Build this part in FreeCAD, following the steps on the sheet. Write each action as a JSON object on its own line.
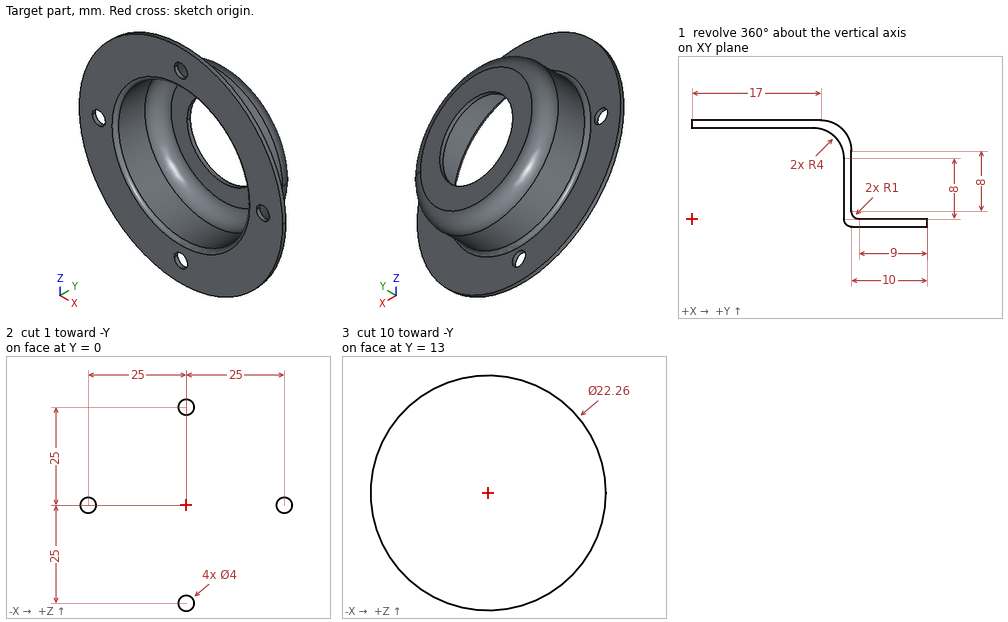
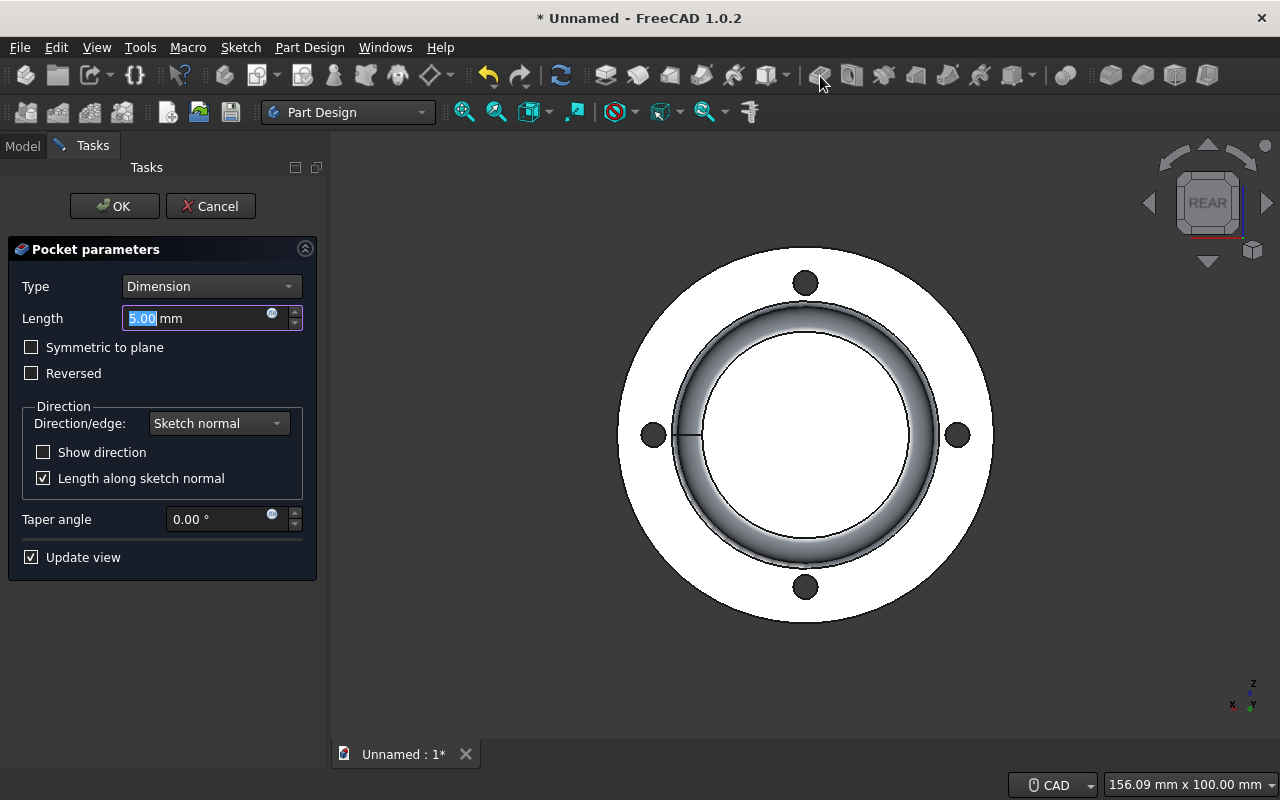
{"action": "type", "text": "1"}
{"action": "key", "text": "Tab"}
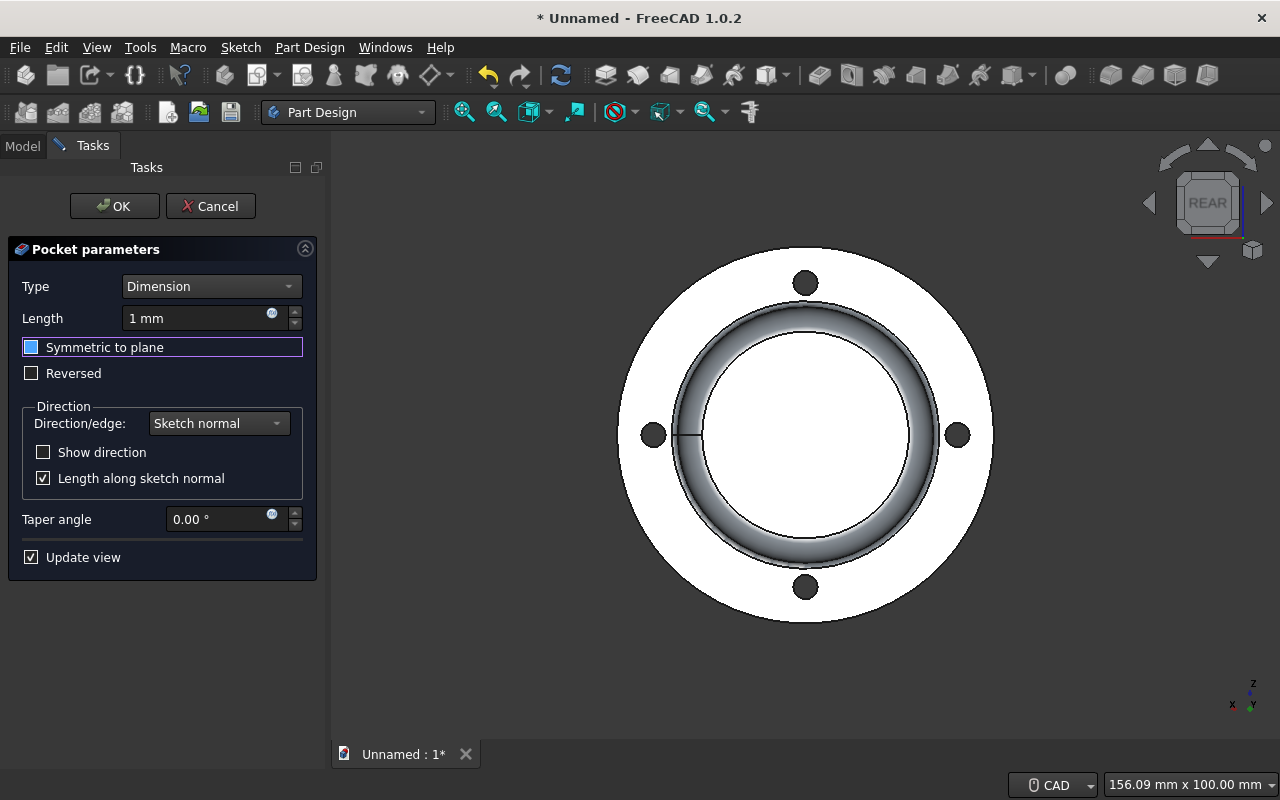
{"action": "left_click", "coordinate": [115, 206]}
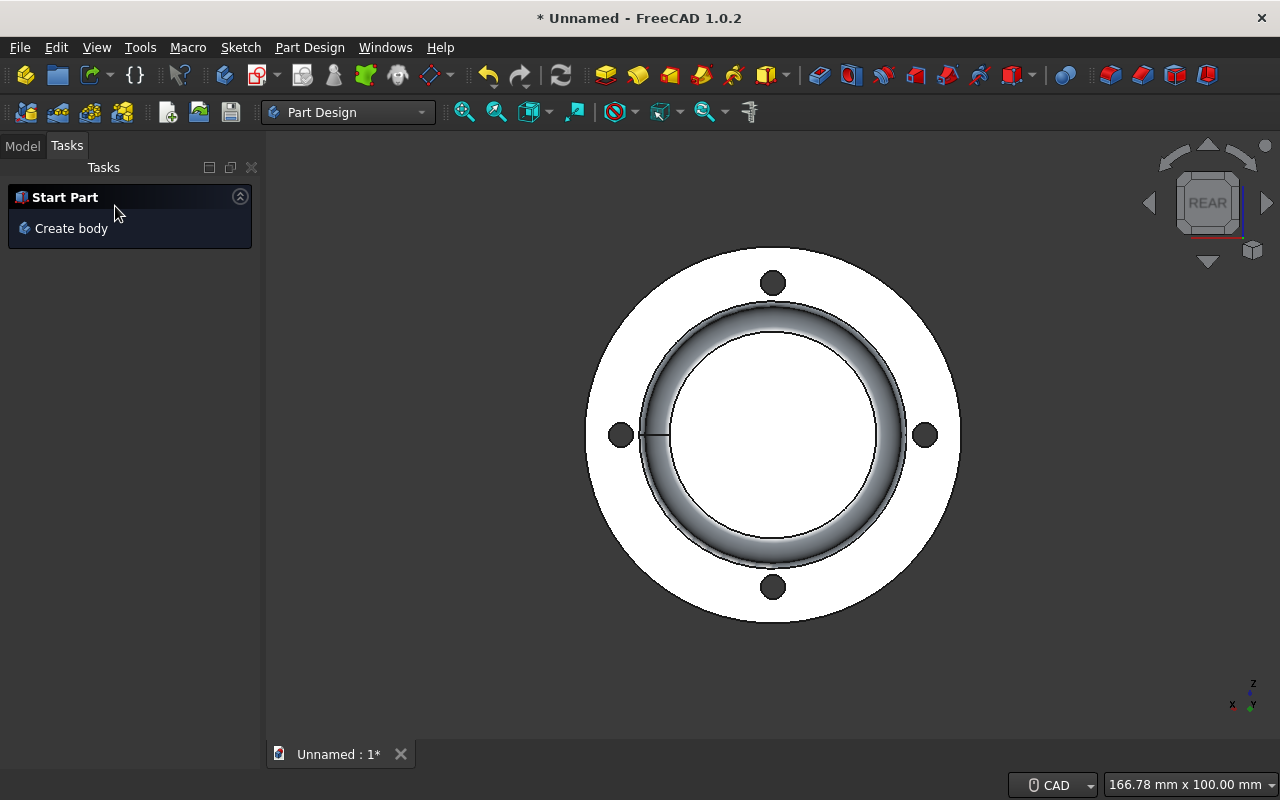
{"action": "left_click", "coordinate": [773, 434]}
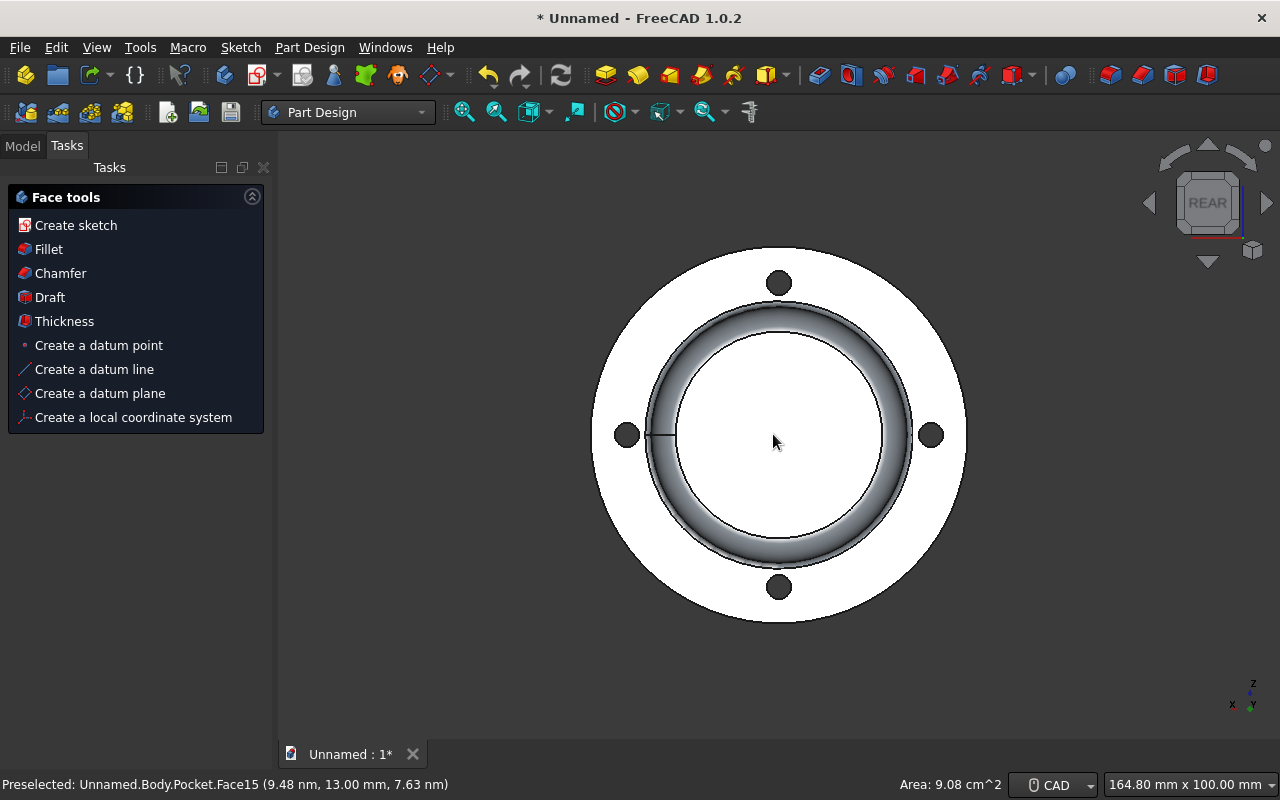
{"action": "left_click", "coordinate": [258, 76]}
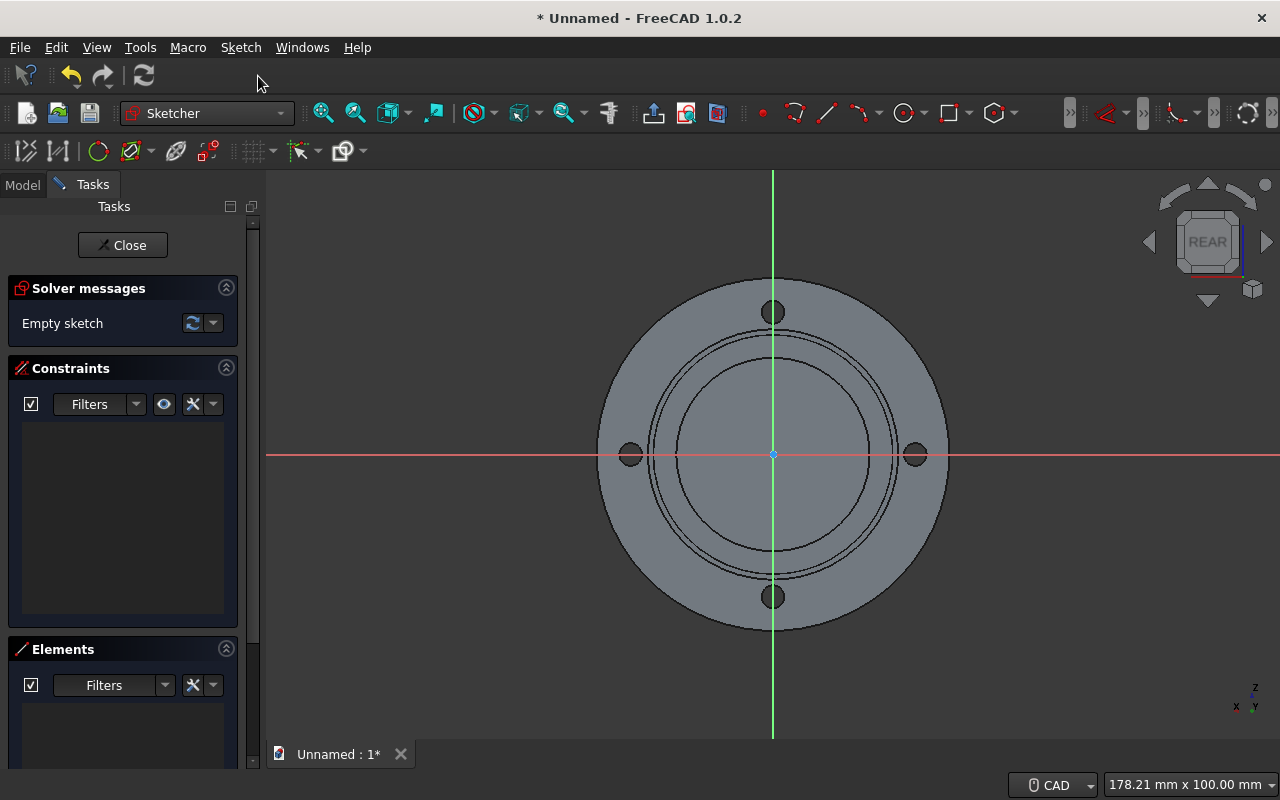
{"action": "scroll", "coordinate": [813, 455], "scroll_direction": "up", "scroll_amount": 5}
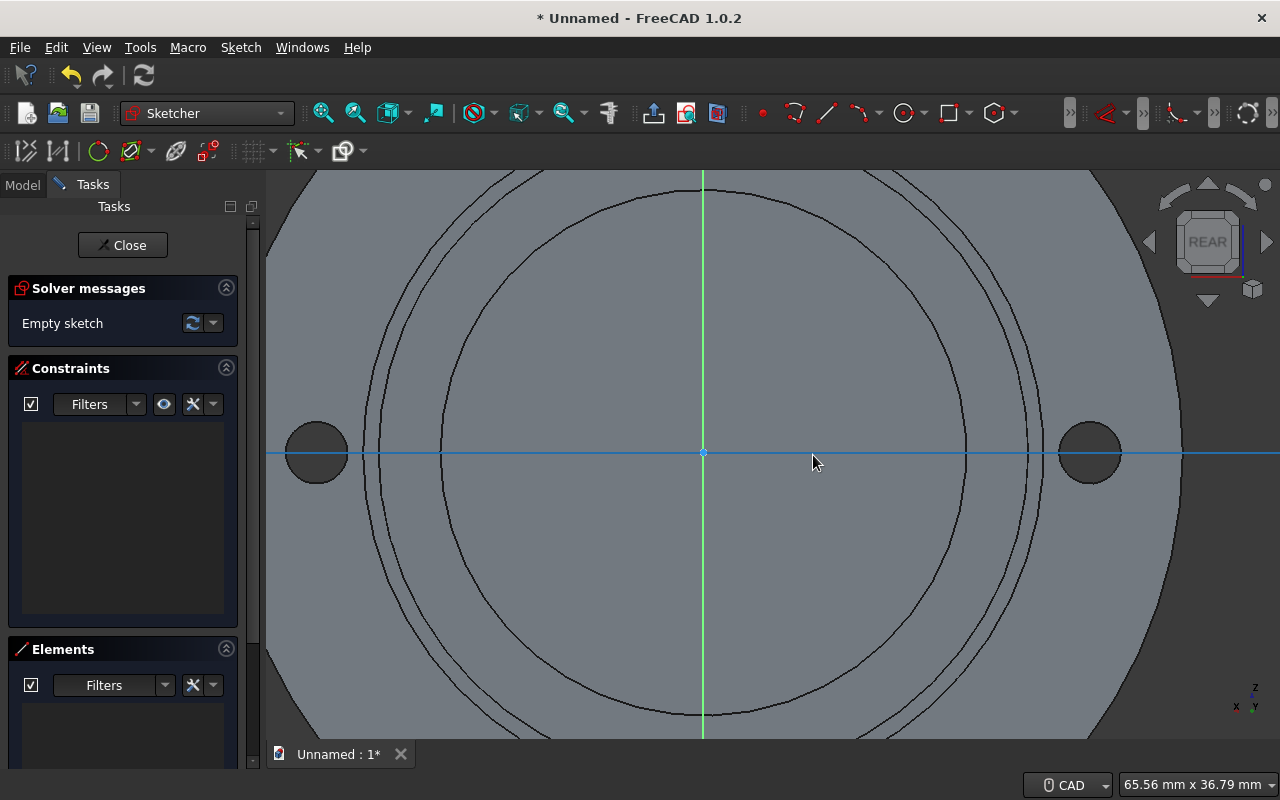
{"action": "key", "text": "g c"}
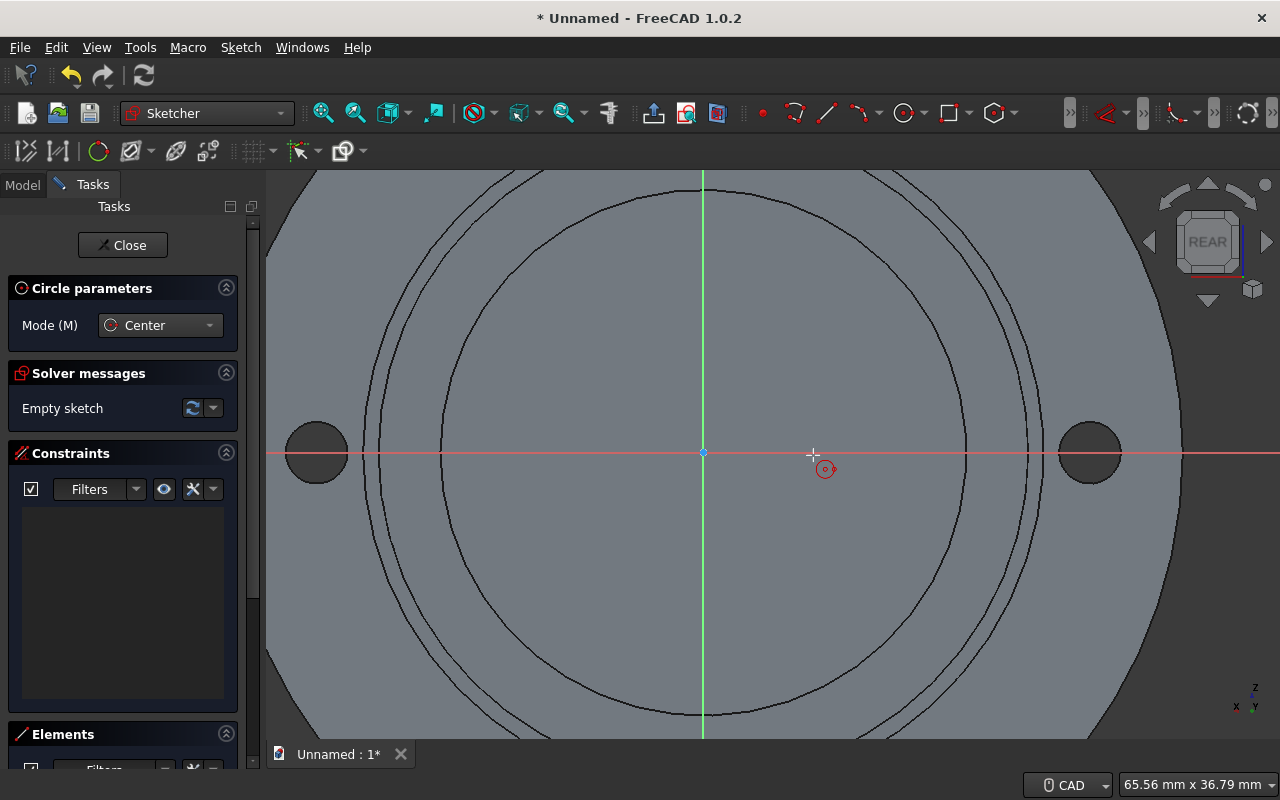
{"action": "left_click", "coordinate": [703, 453]}
{"action": "left_click", "coordinate": [825, 331]}
{"action": "key", "text": "Escape"}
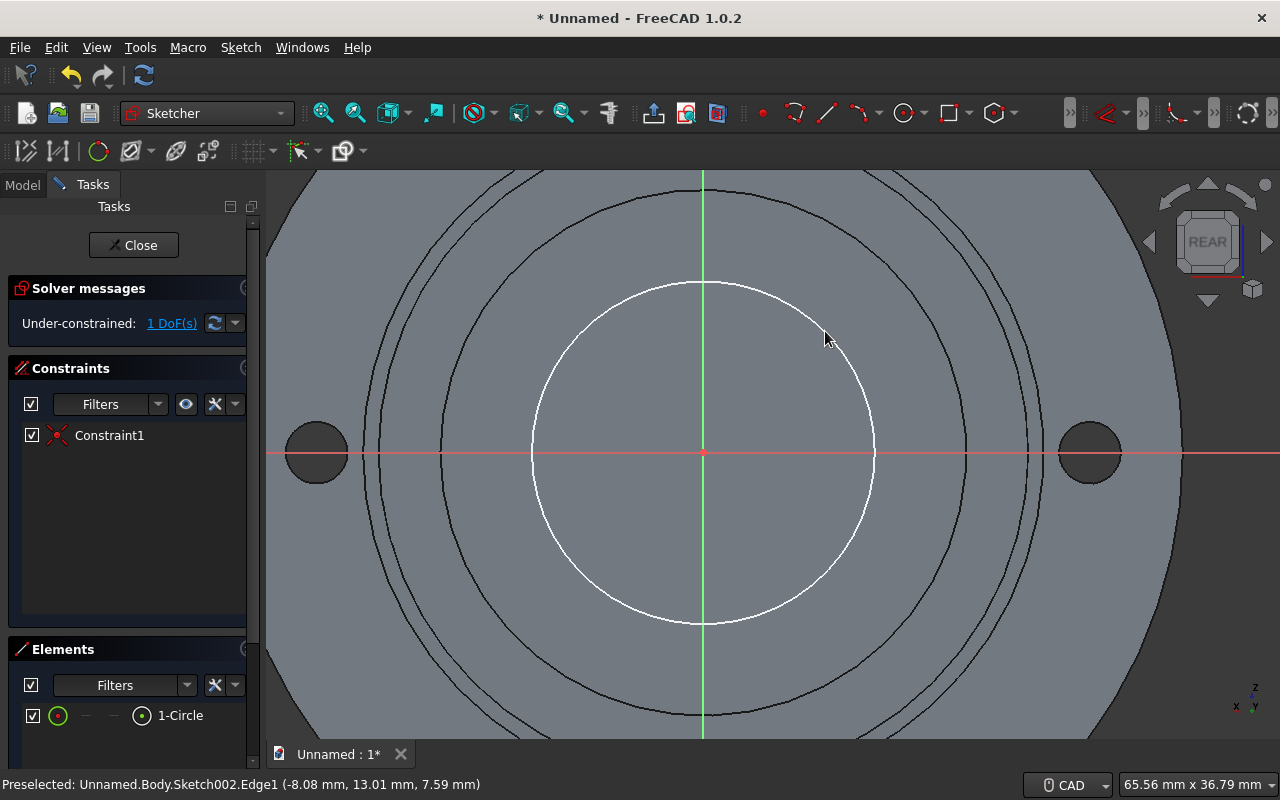
{"action": "key", "text": "d"}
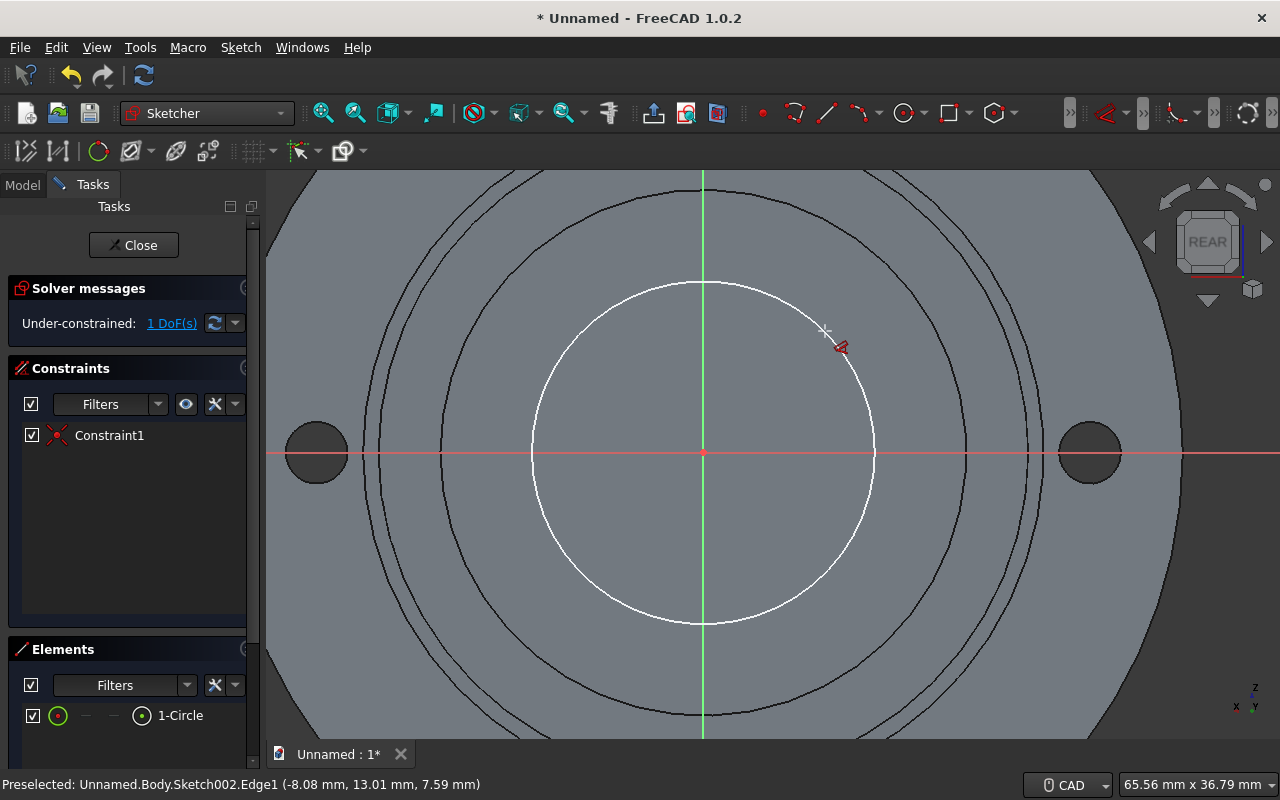
{"action": "left_click", "coordinate": [824, 331]}
{"action": "left_click", "coordinate": [847, 308]}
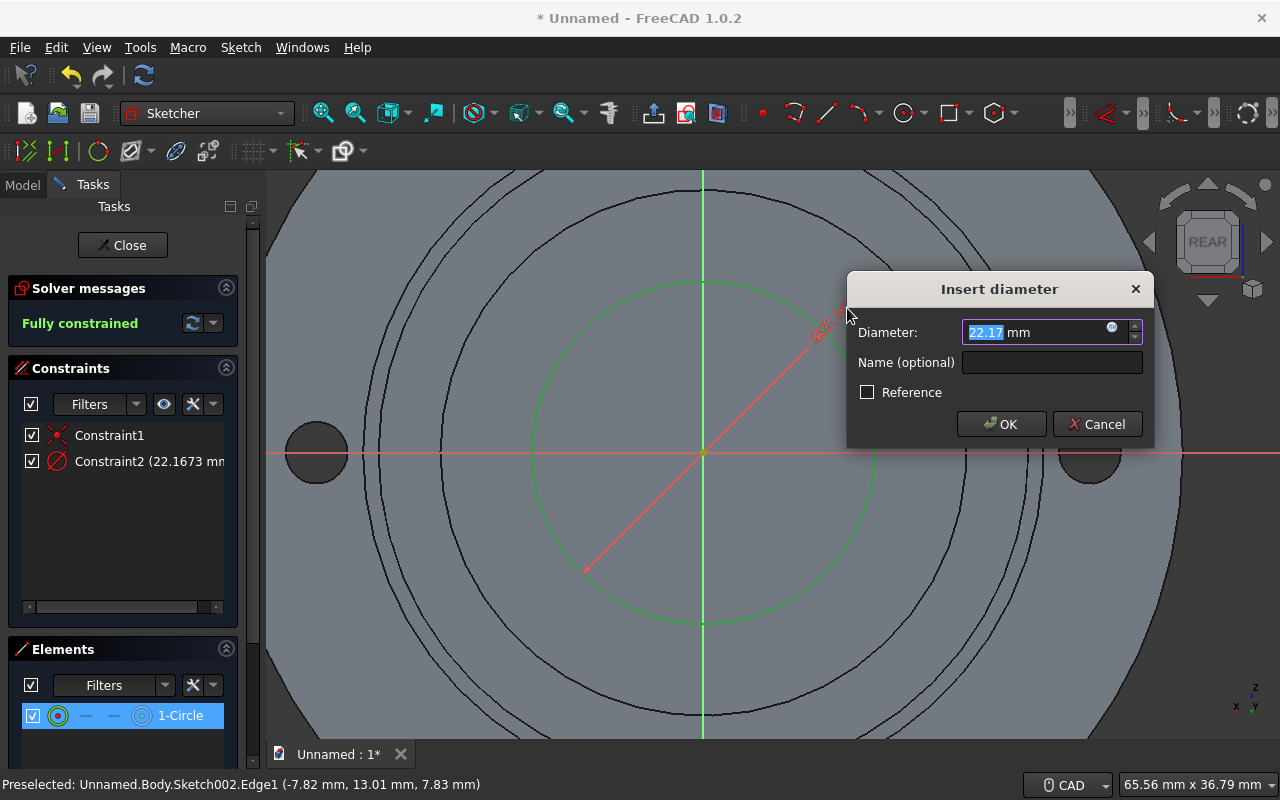
{"action": "type", "text": "22.26"}
{"action": "key", "text": "Return"}
{"action": "key", "text": "Escape"}